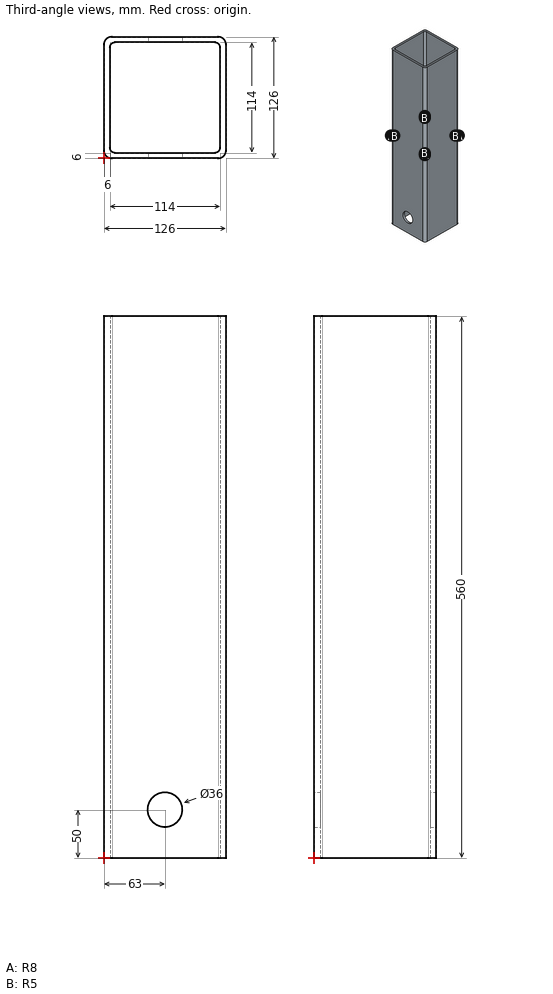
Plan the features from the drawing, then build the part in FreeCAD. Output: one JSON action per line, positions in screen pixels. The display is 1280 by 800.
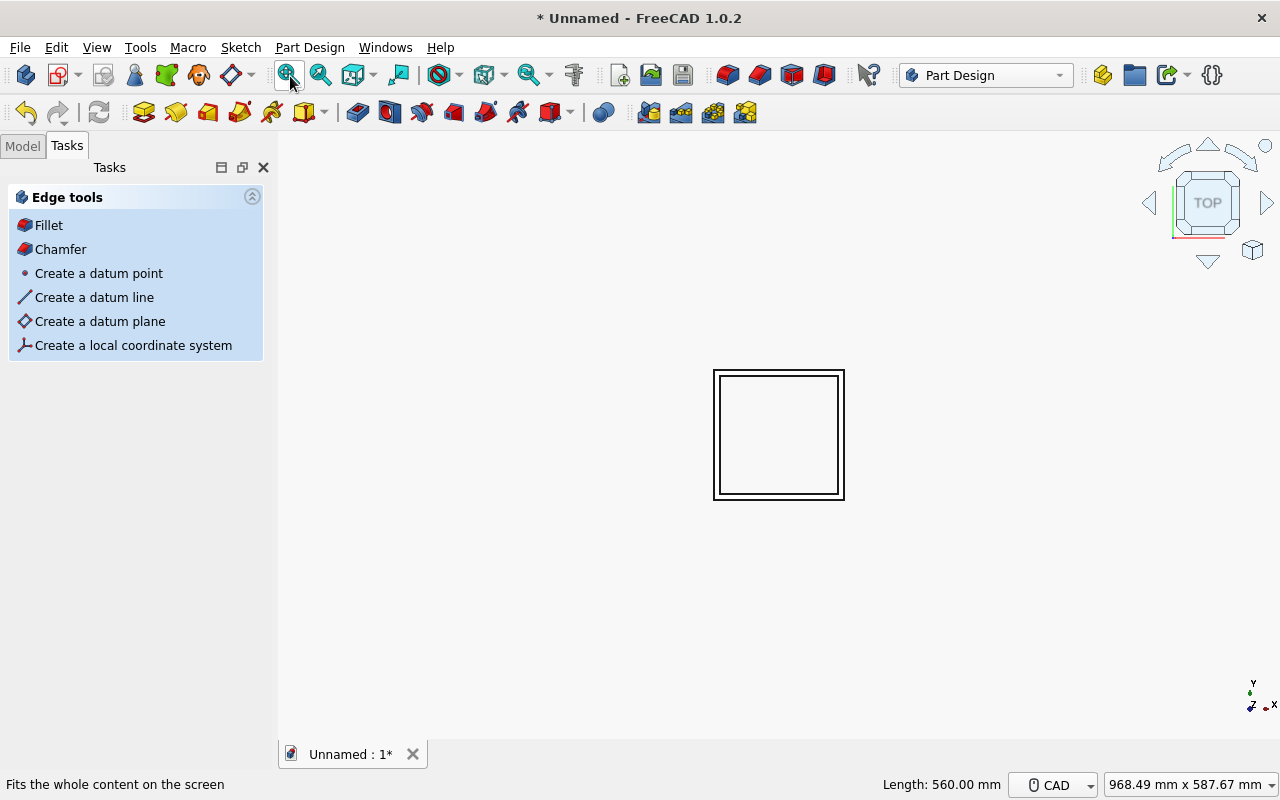
{"action": "key", "text": "1"}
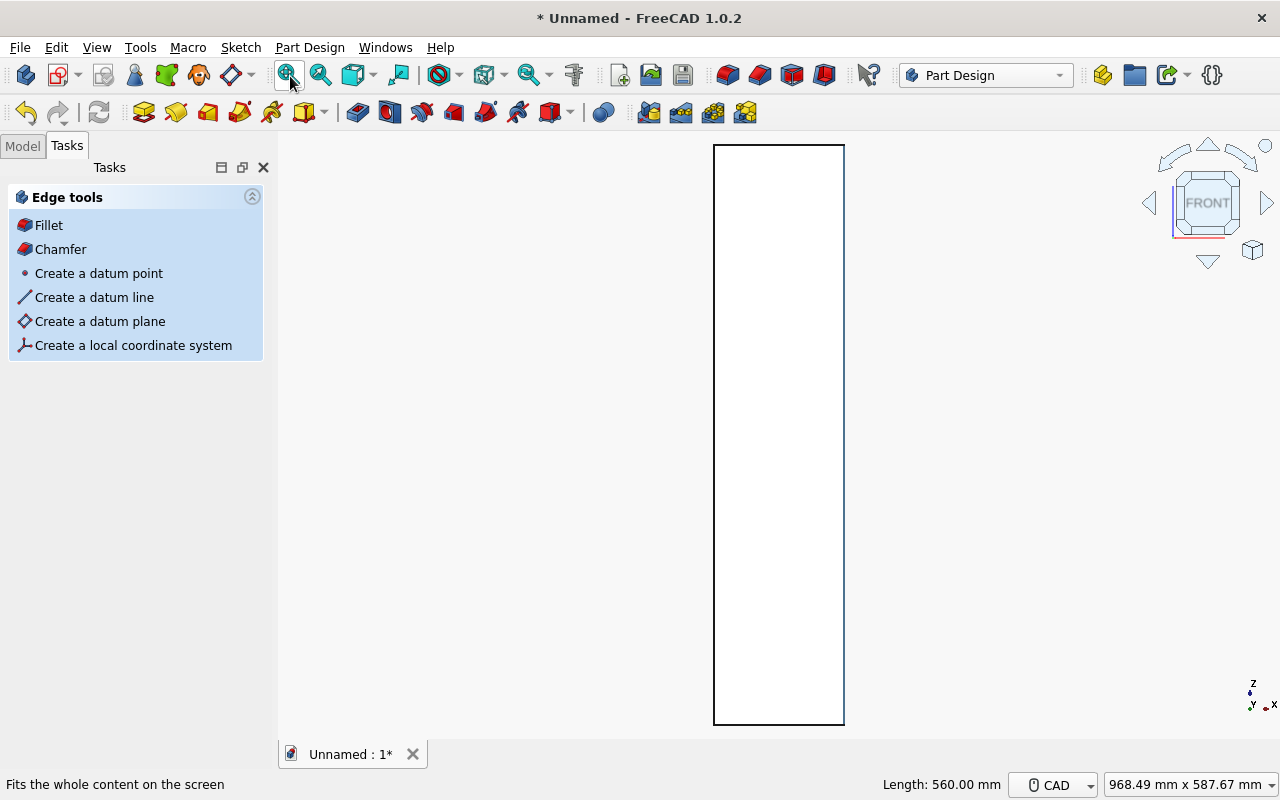
{"action": "left_click", "coordinate": [714, 434], "text": "ctrl"}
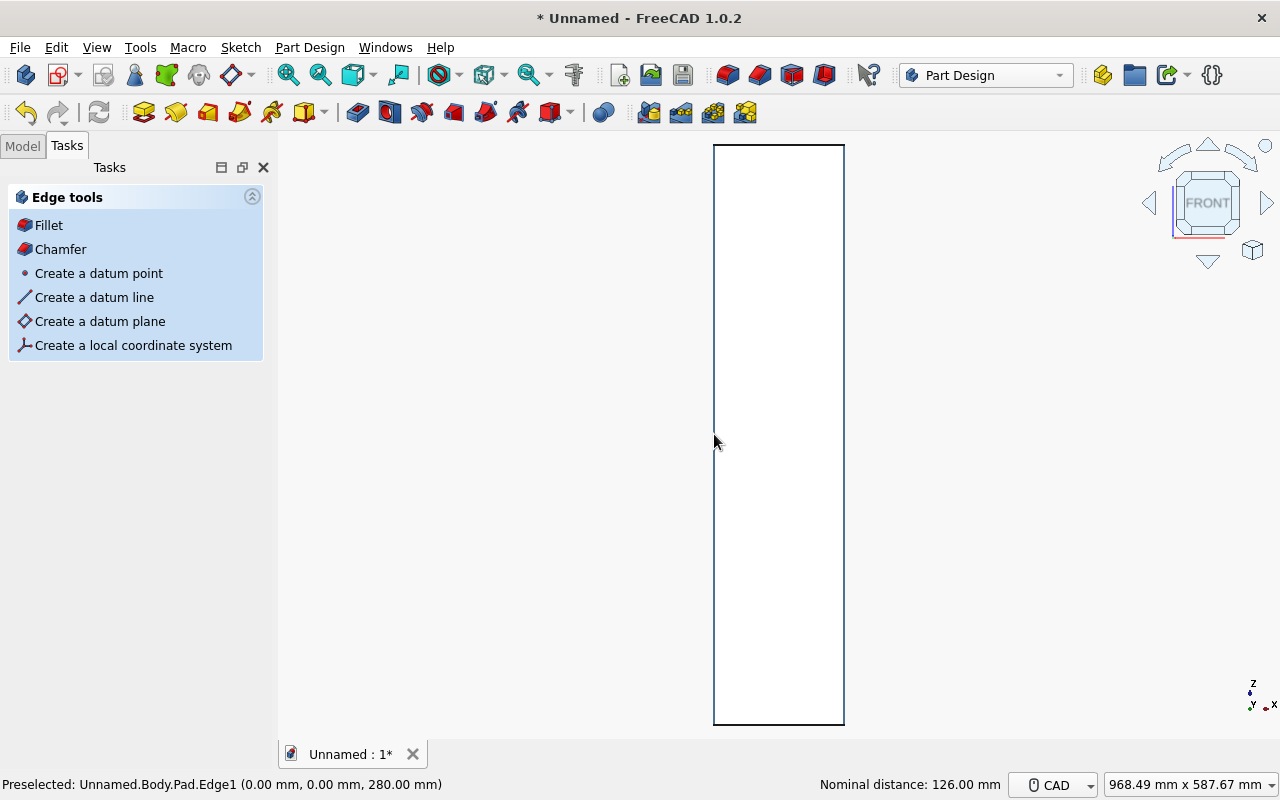
{"action": "key", "text": "3"}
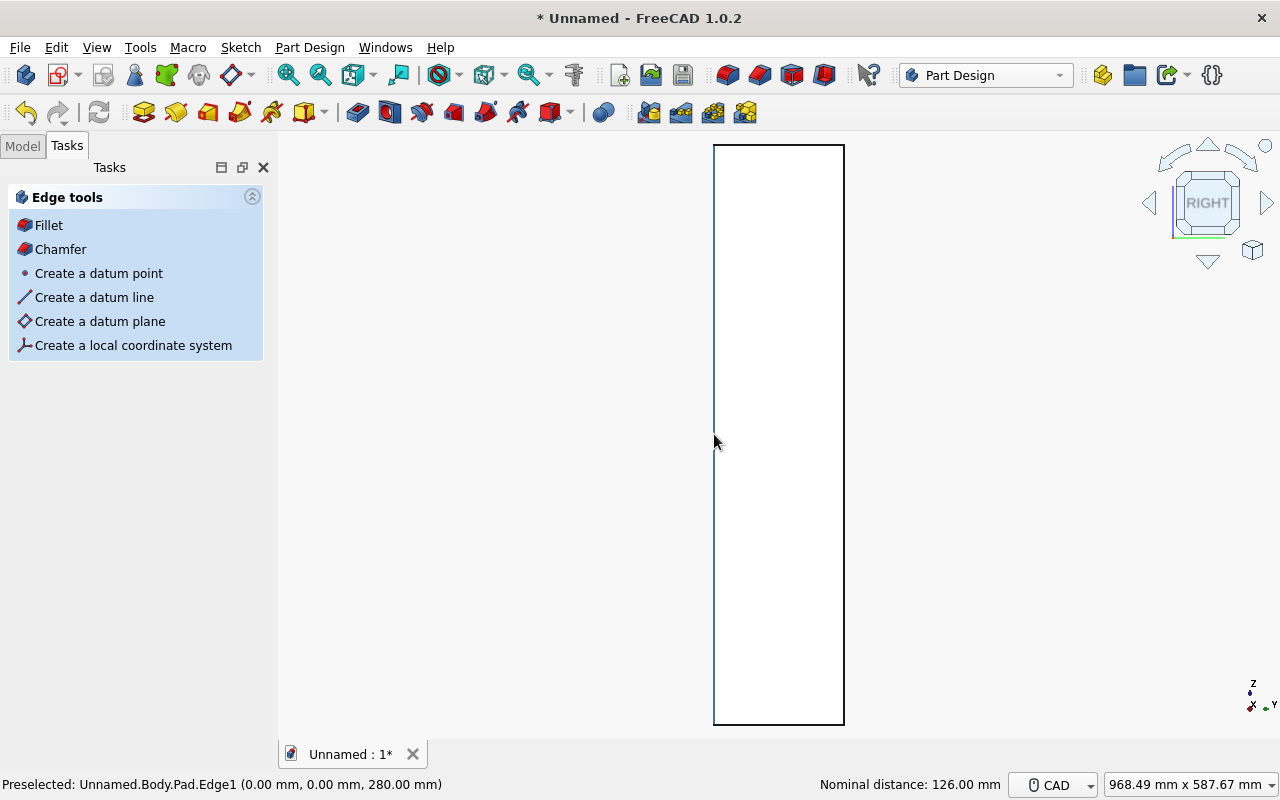
{"action": "left_click", "coordinate": [844, 434], "text": "ctrl"}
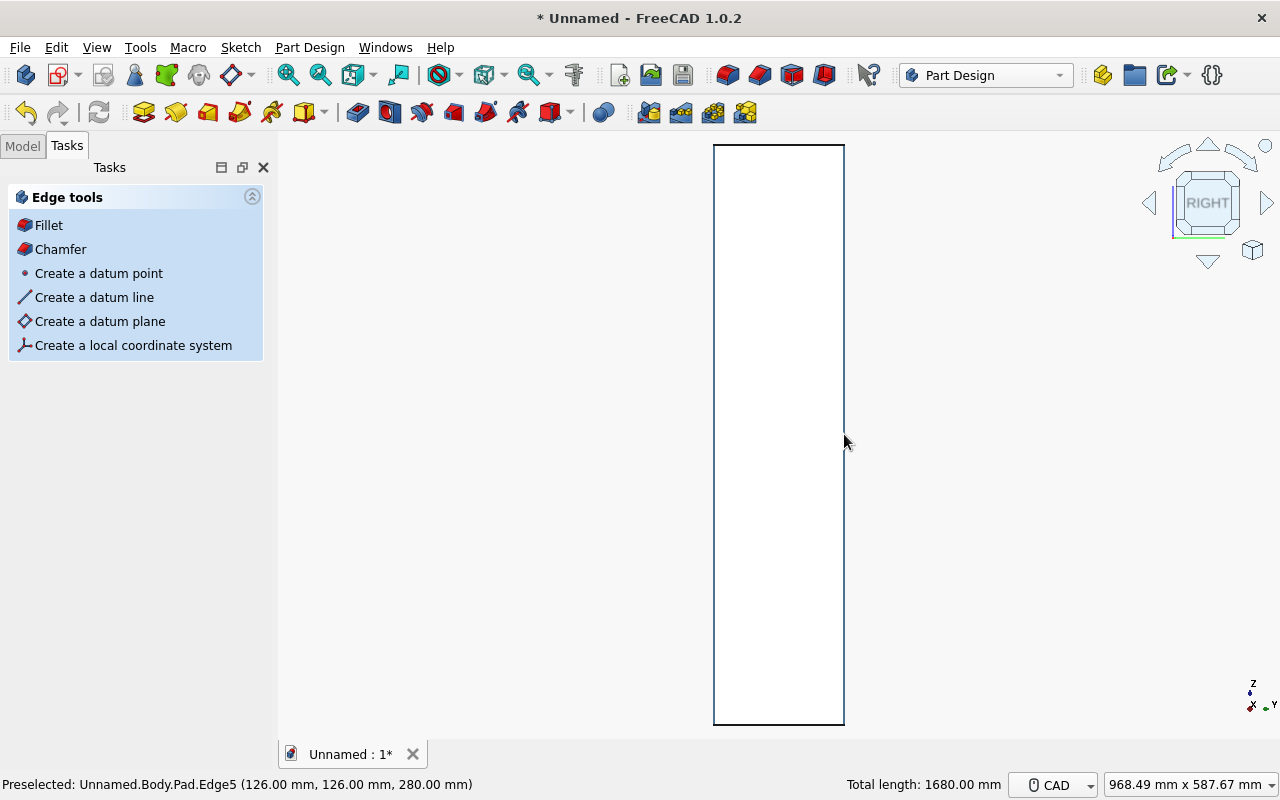
{"action": "key", "text": "5"}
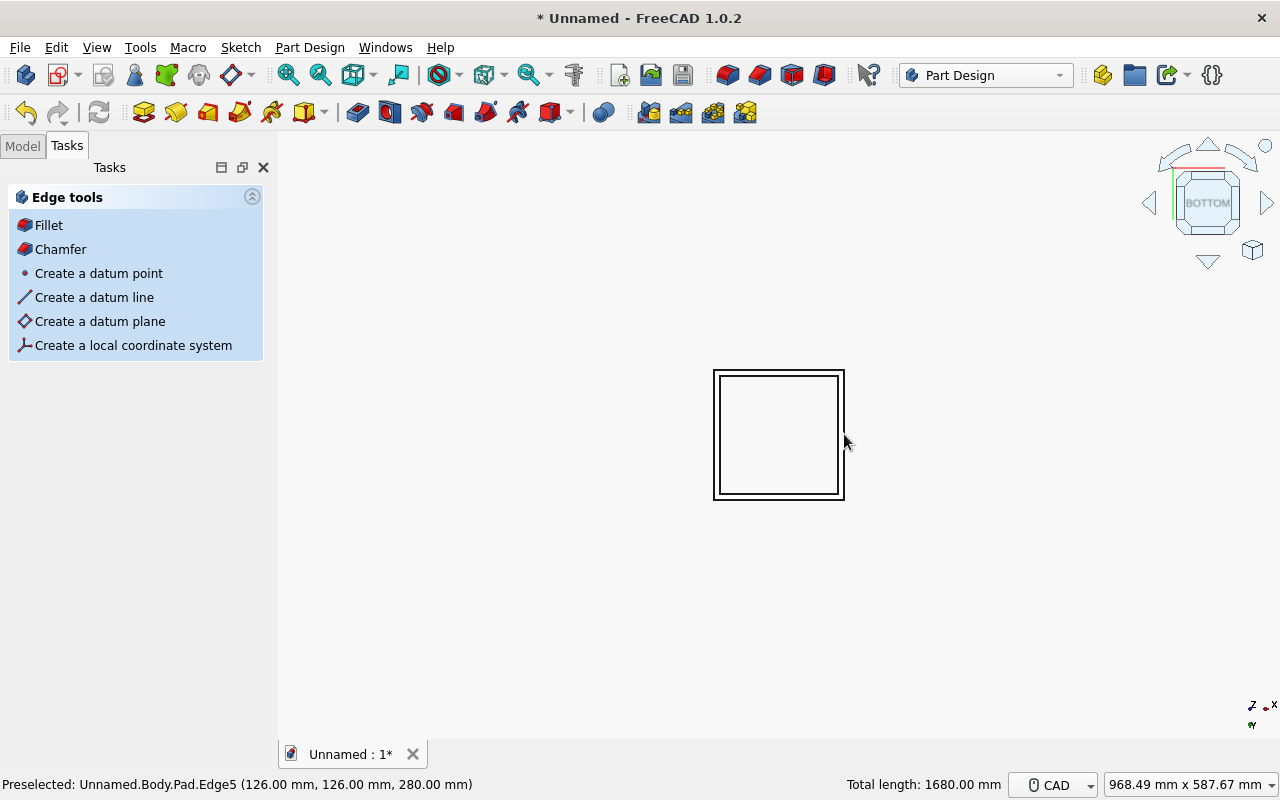
{"action": "left_click", "coordinate": [290, 76]}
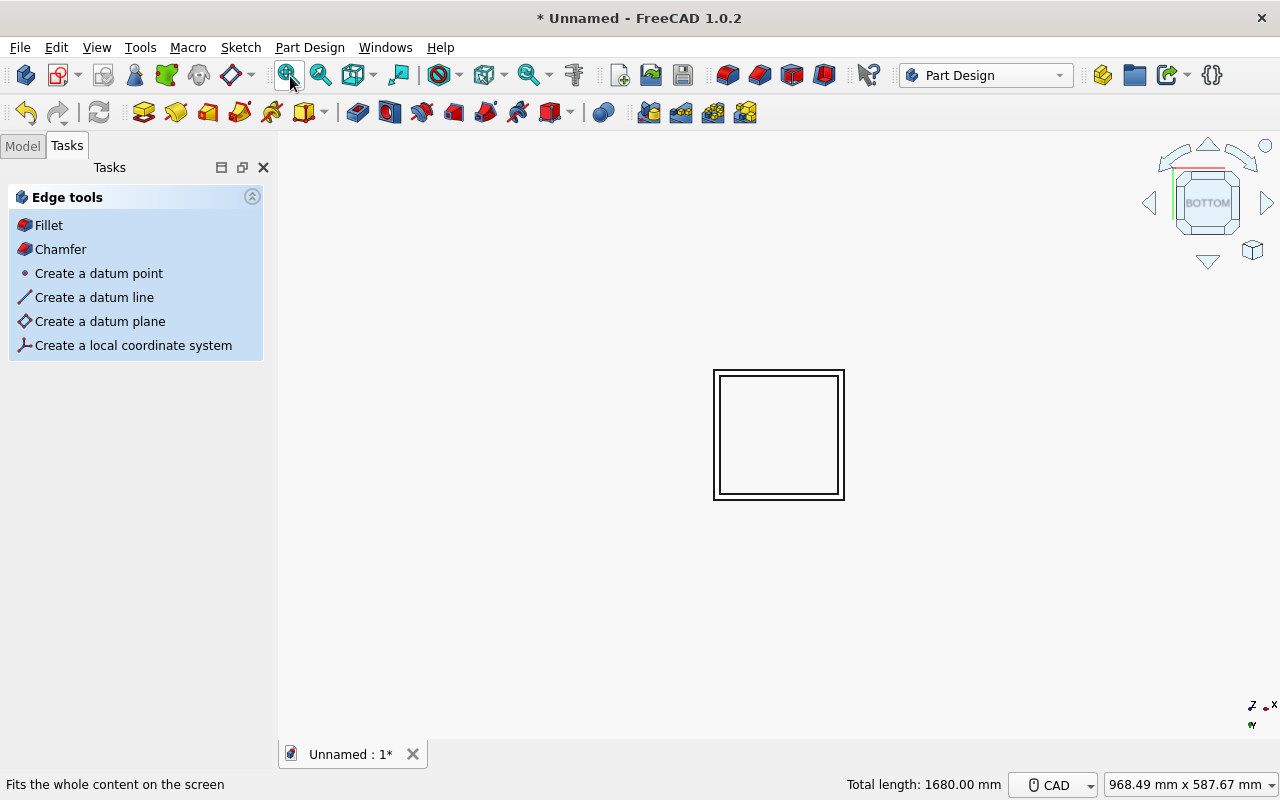
{"action": "key", "text": "4"}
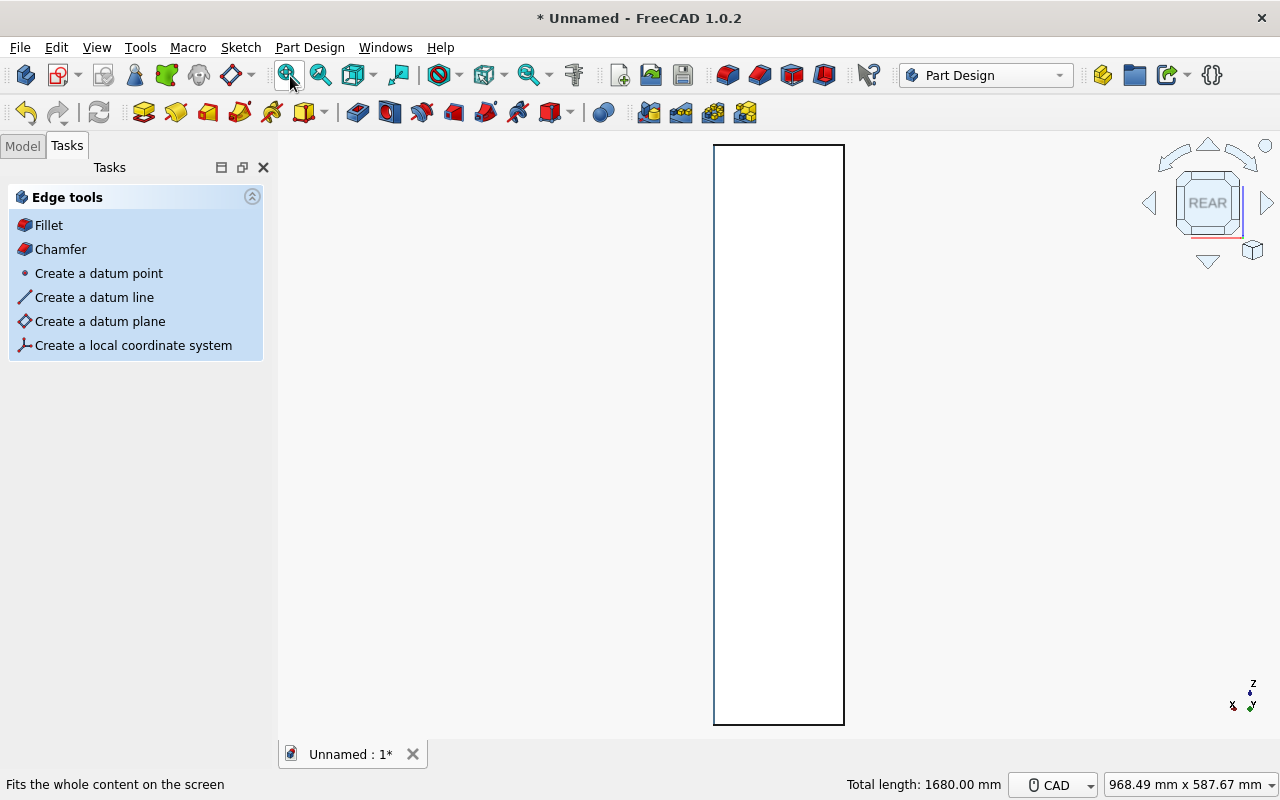
{"action": "left_click", "coordinate": [844, 434], "text": "ctrl"}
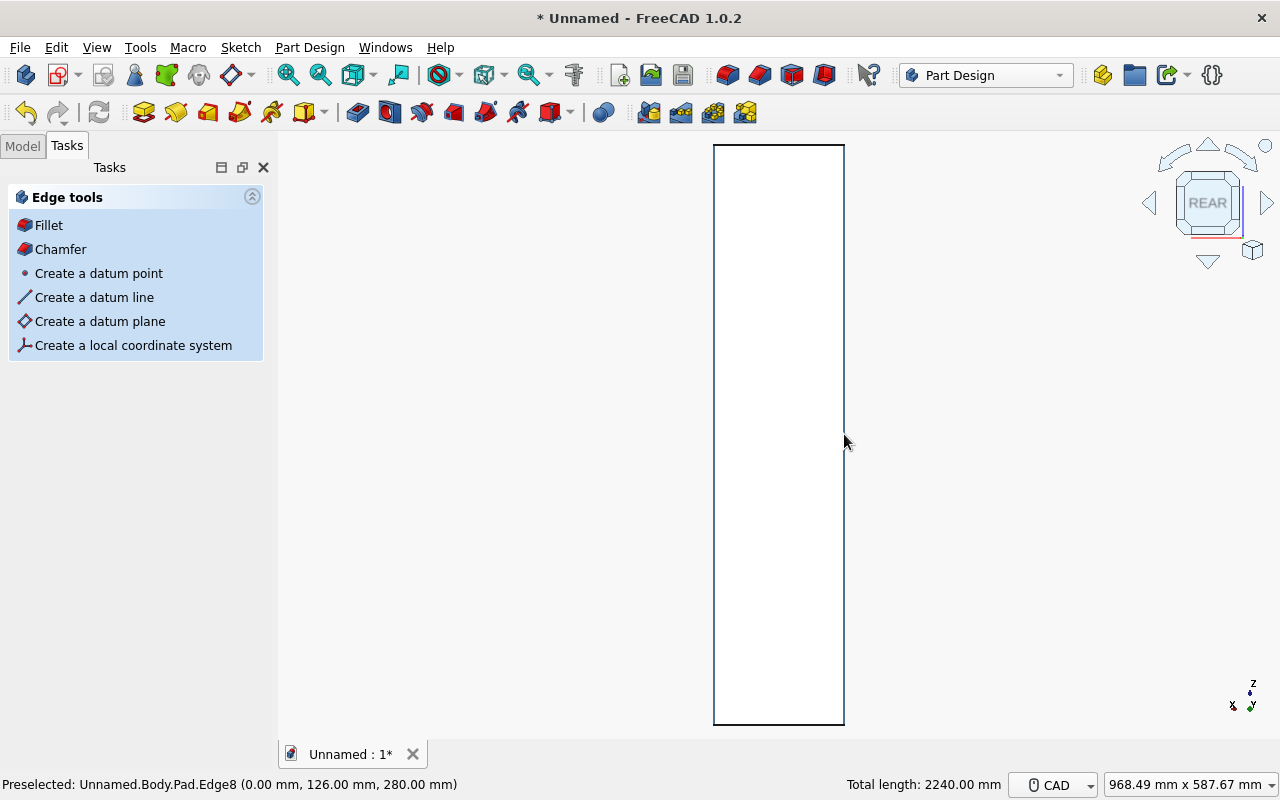
{"action": "left_click", "coordinate": [728, 76]}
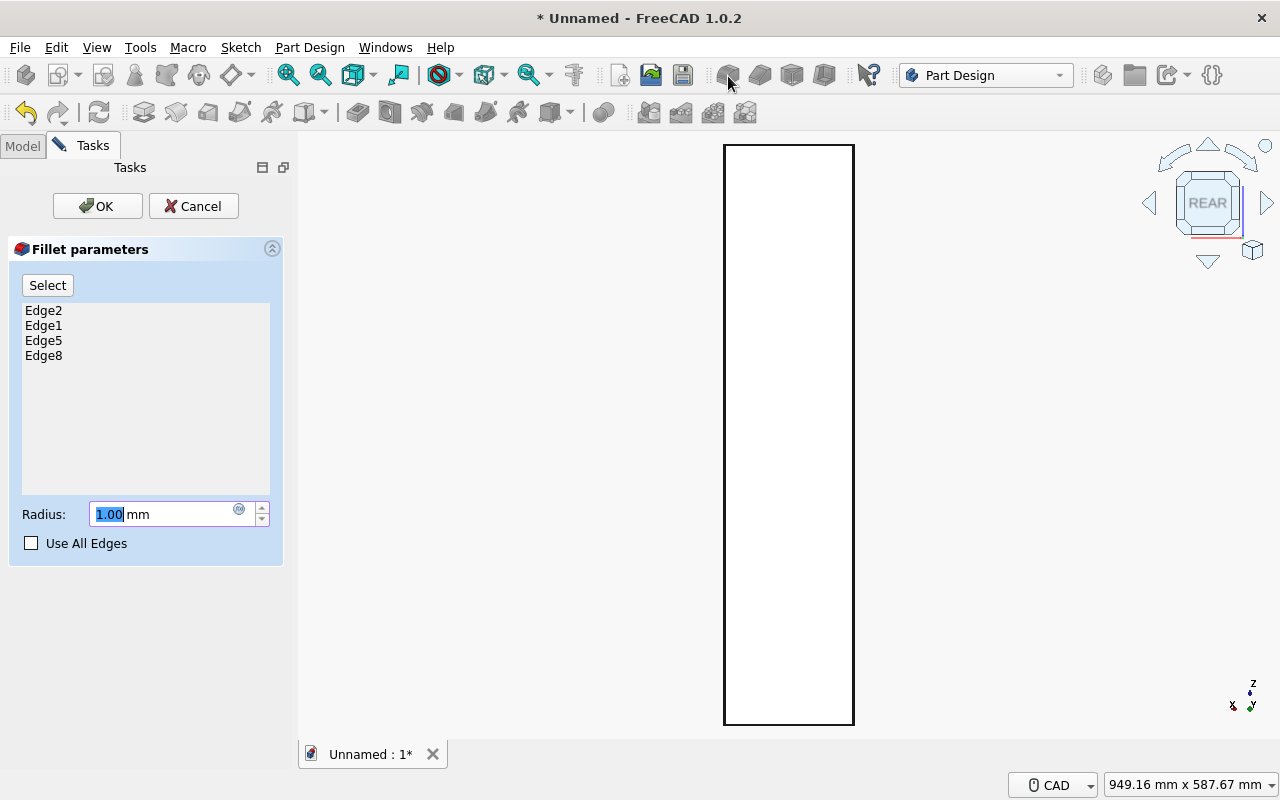
{"action": "type", "text": "8"}
{"action": "key", "text": "Tab"}